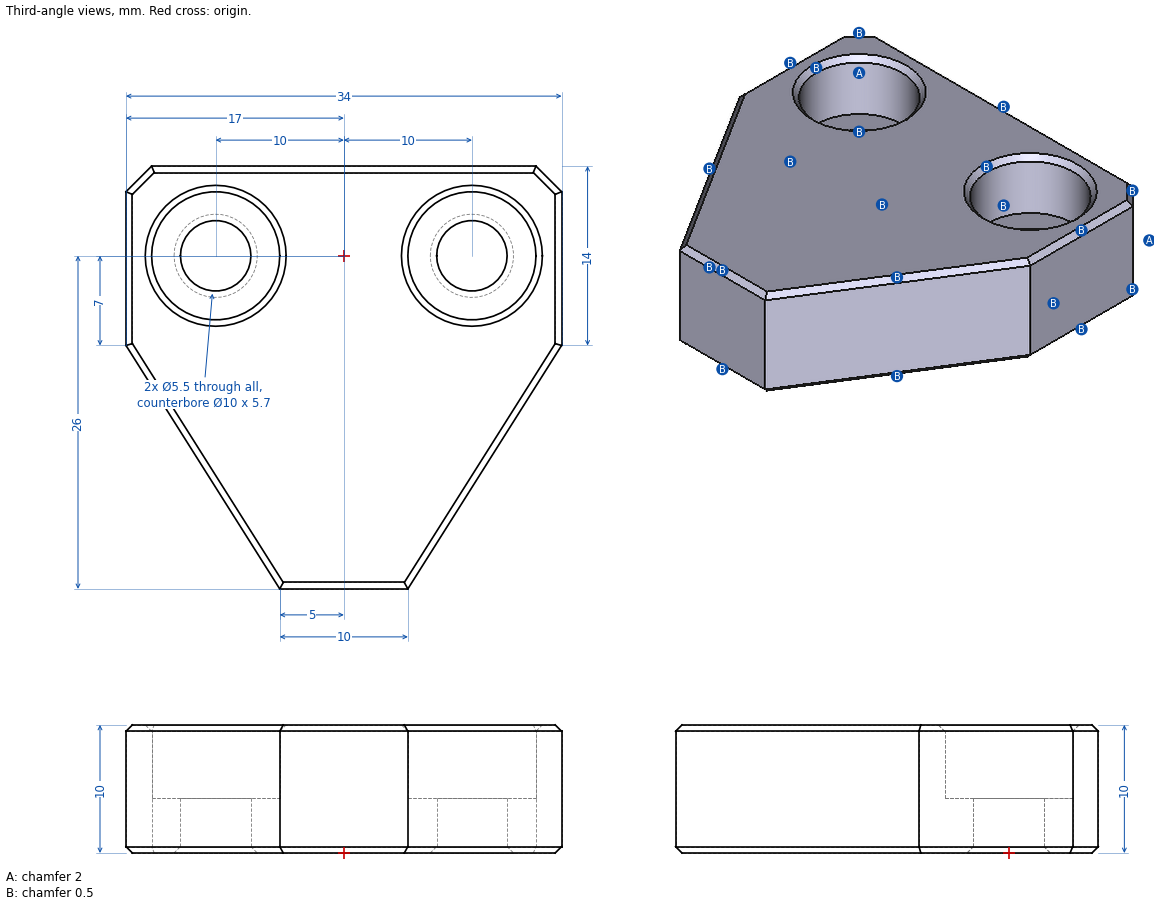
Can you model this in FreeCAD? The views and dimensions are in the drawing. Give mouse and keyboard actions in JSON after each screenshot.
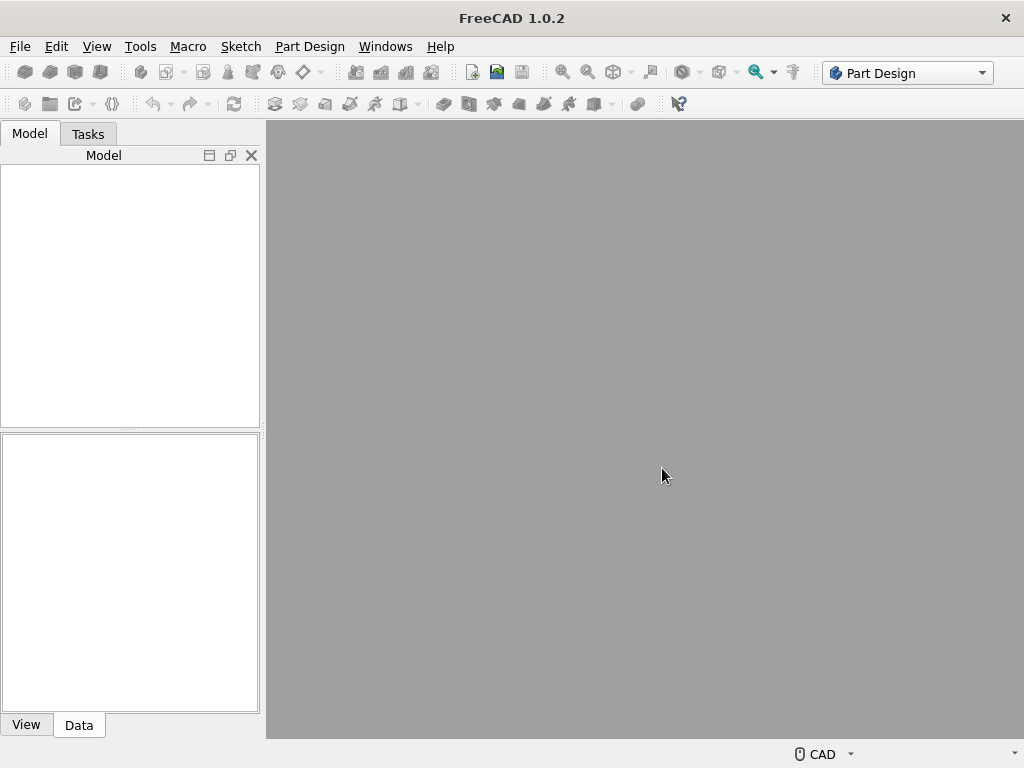
{"action": "left_click", "coordinate": [472, 72]}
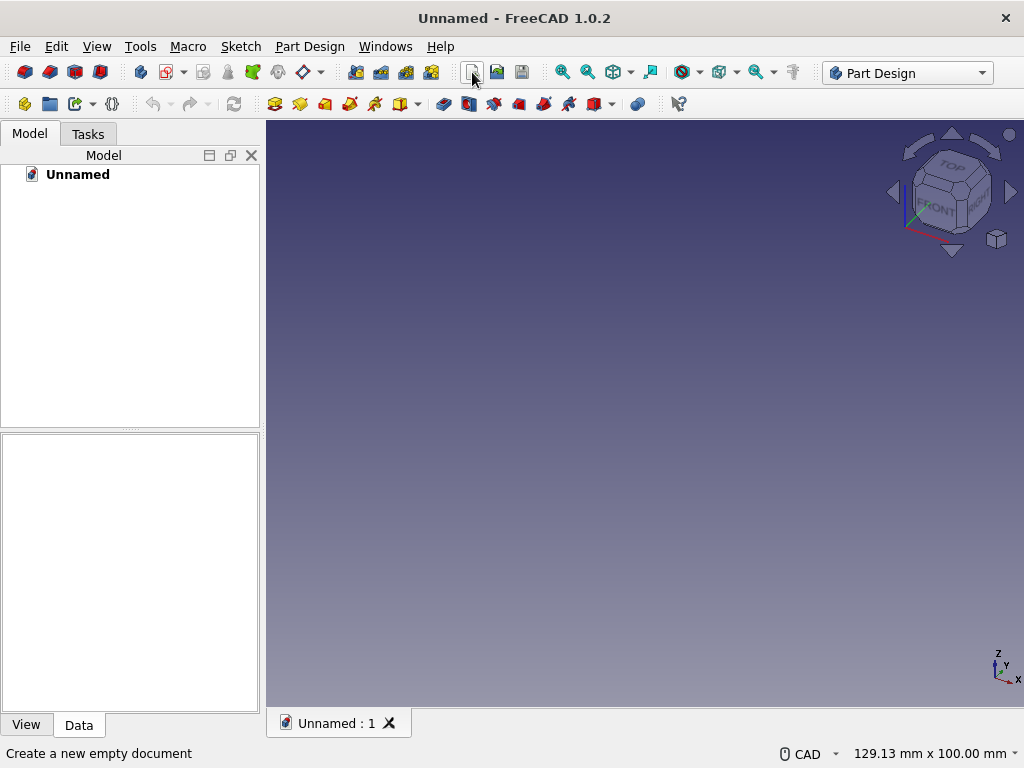
{"action": "left_click", "coordinate": [166, 72]}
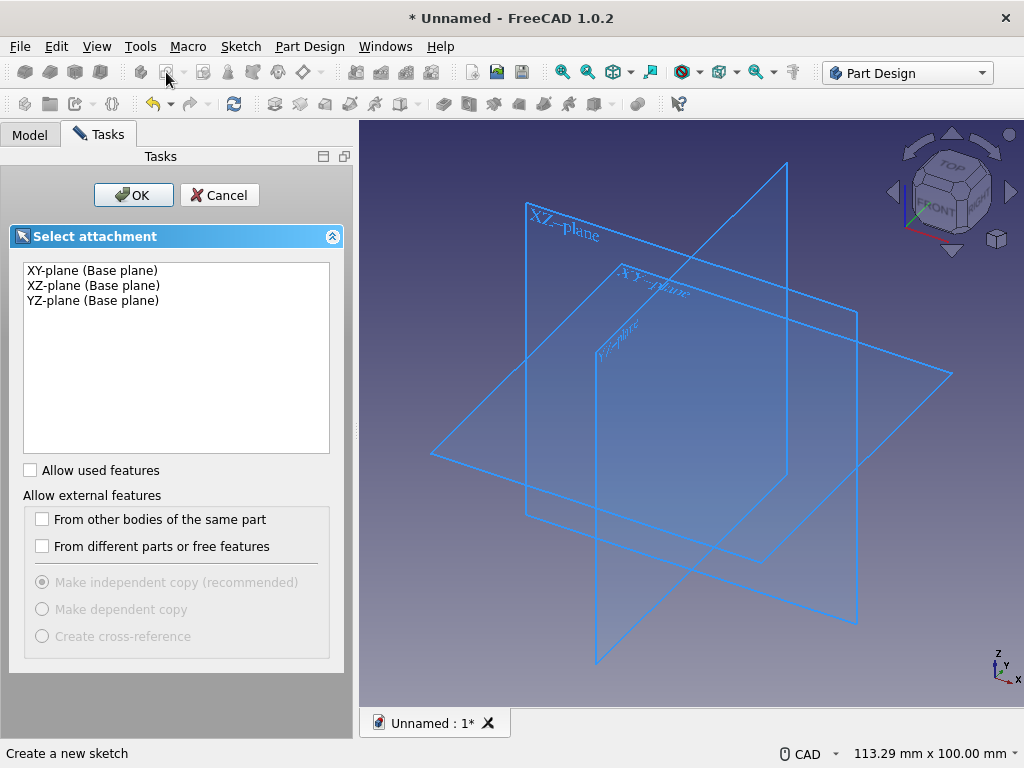
{"action": "left_click", "coordinate": [84, 270]}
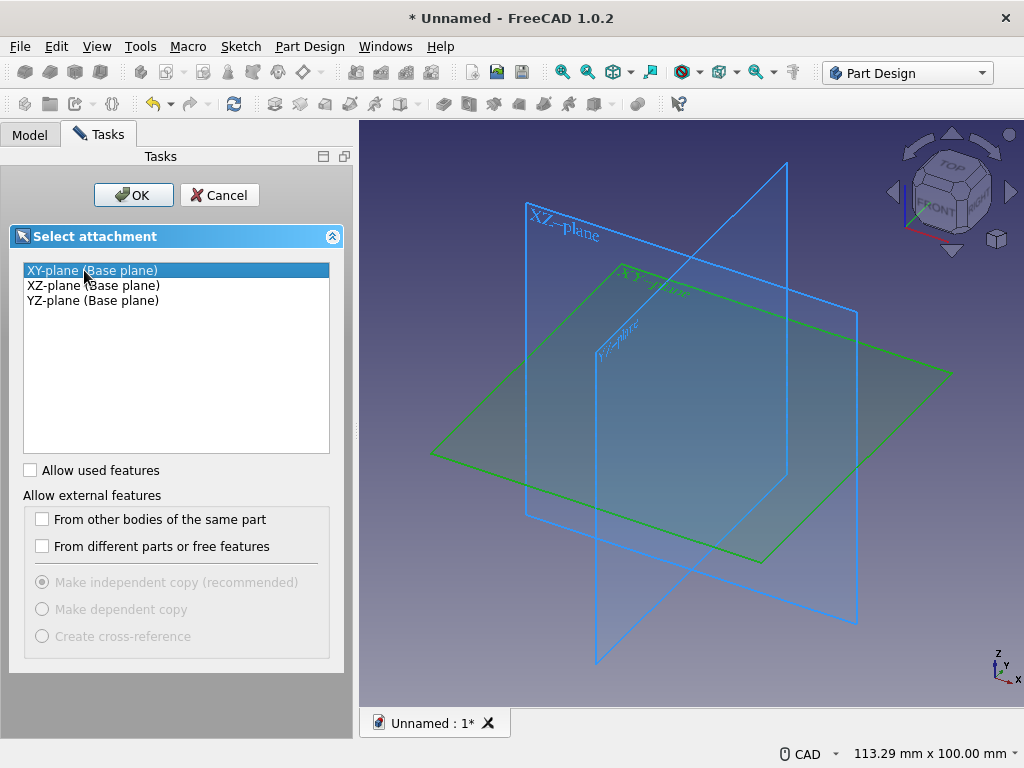
{"action": "left_click", "coordinate": [134, 195]}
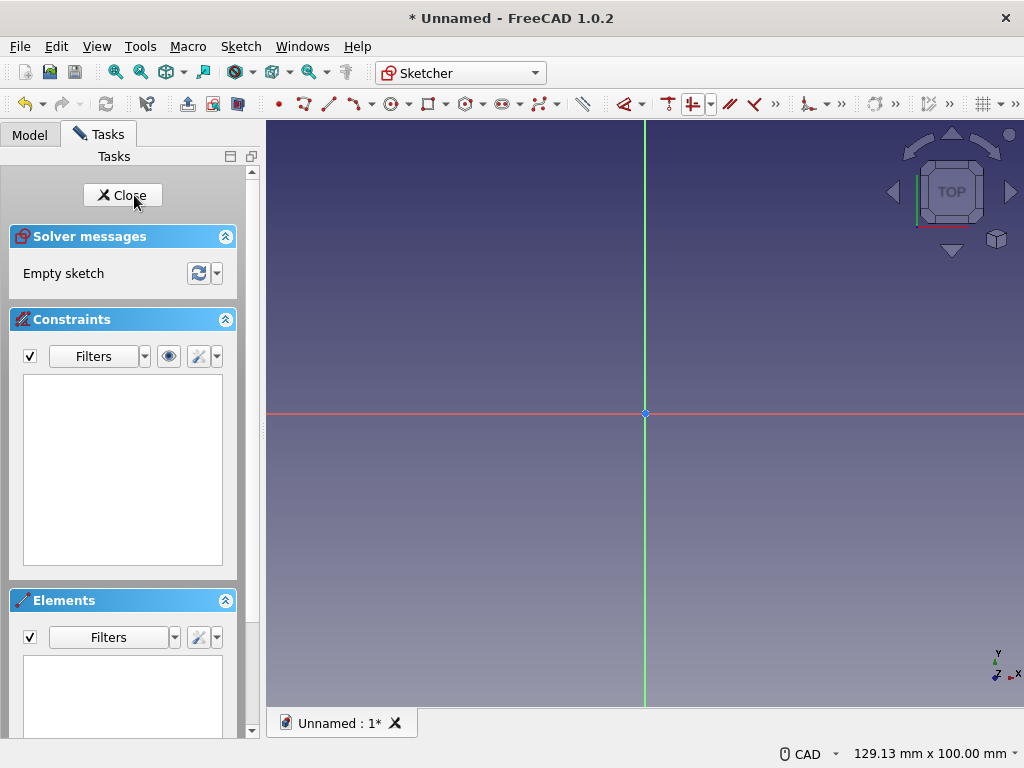
{"action": "scroll", "coordinate": [728, 414], "scroll_direction": "up", "scroll_amount": 3}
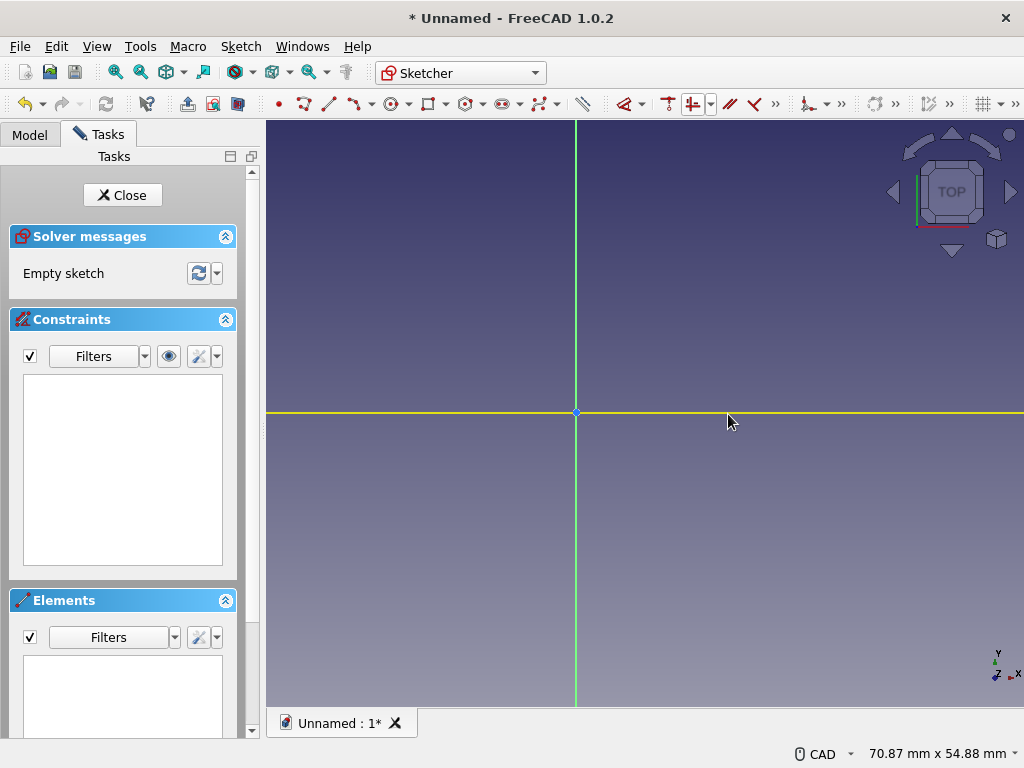
{"action": "key", "text": "g v"}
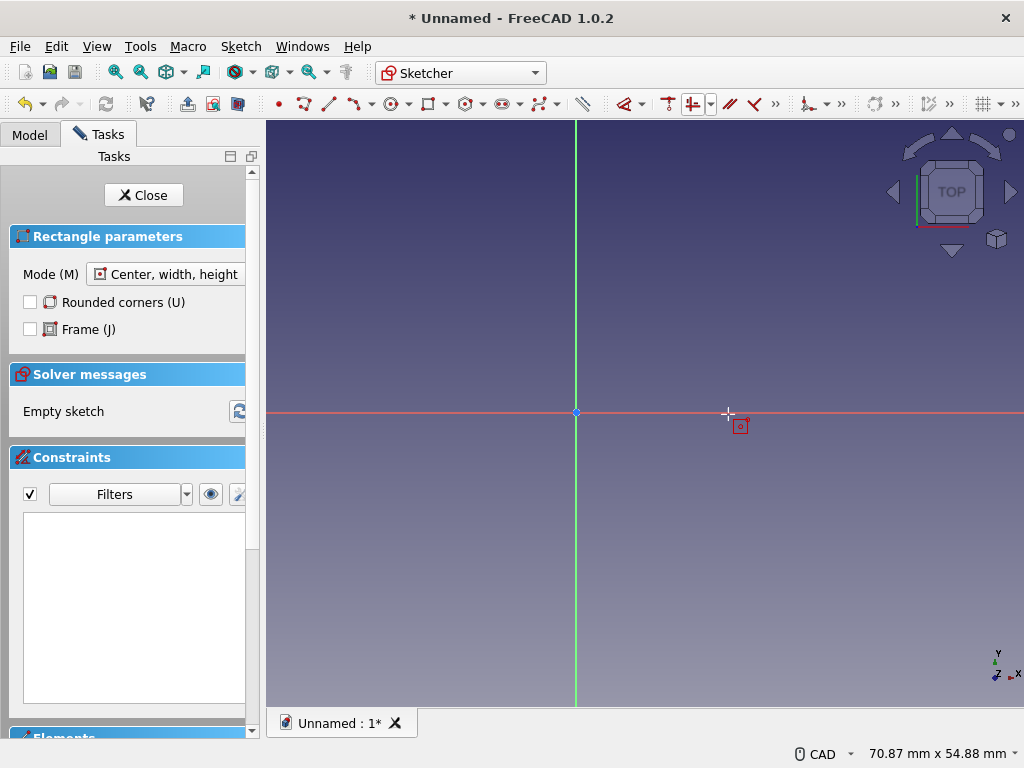
{"action": "left_click", "coordinate": [576, 413]}
{"action": "mouse_move", "coordinate": [758, 338]}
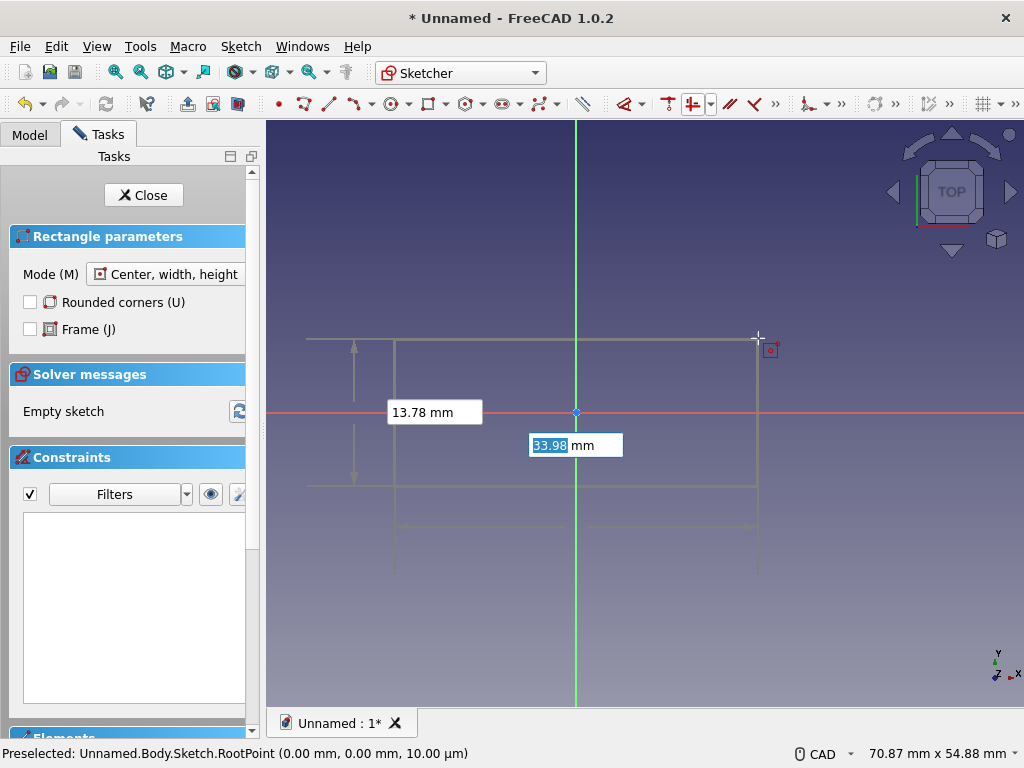
{"action": "type", "text": "34"}
{"action": "key", "text": "Tab"}
{"action": "type", "text": "14"}
{"action": "key", "text": "Return"}
{"action": "key", "text": "Escape"}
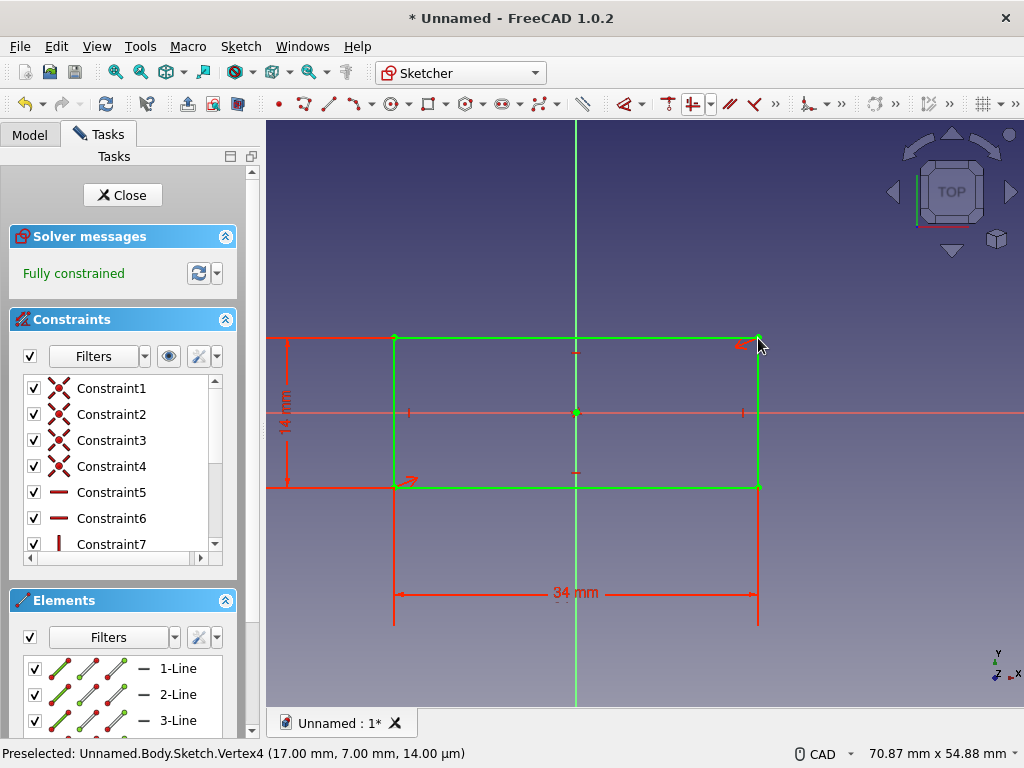
{"action": "left_click", "coordinate": [123, 195]}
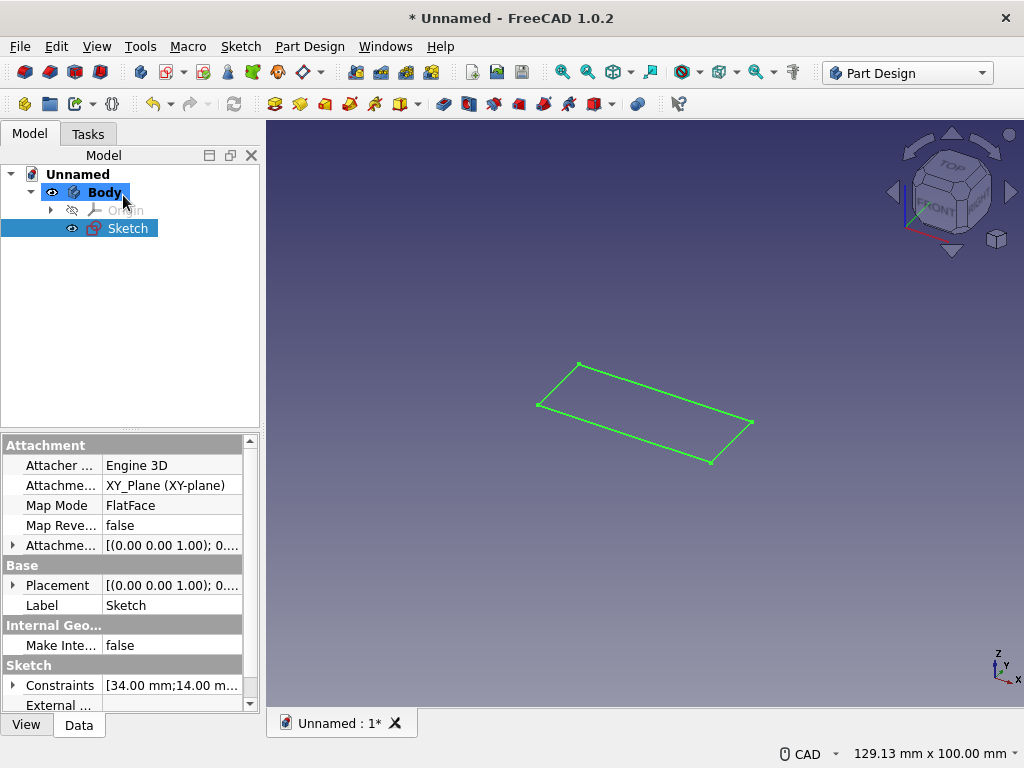
{"action": "left_click", "coordinate": [275, 104]}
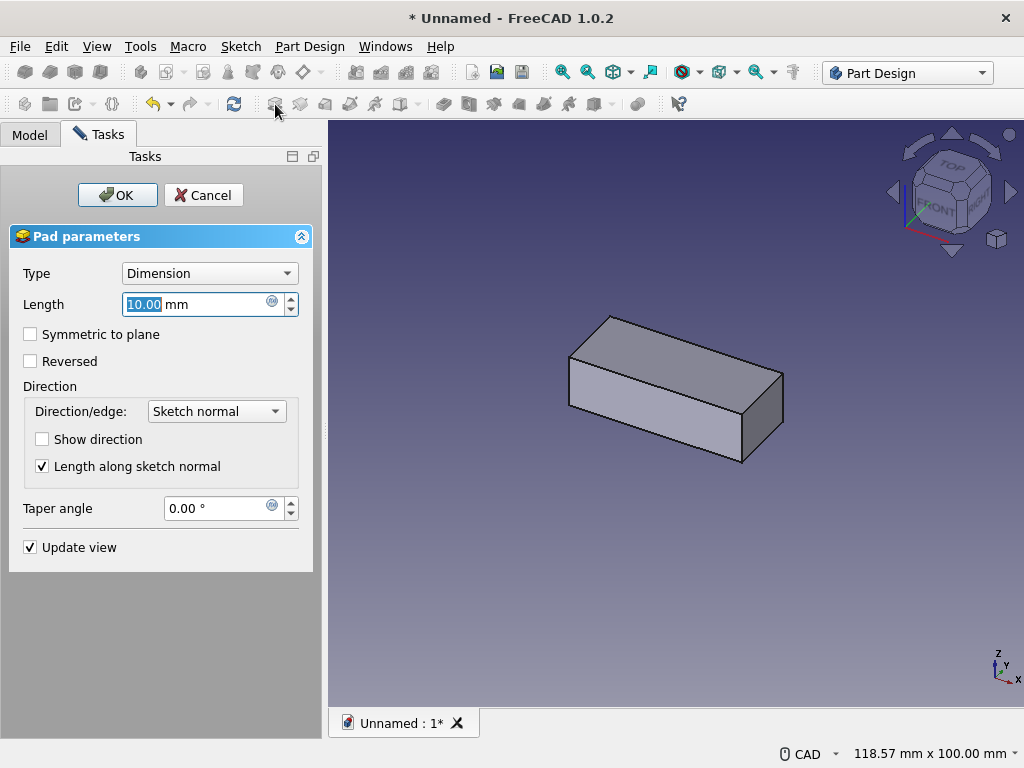
{"action": "type", "text": "10"}
{"action": "key", "text": "Tab"}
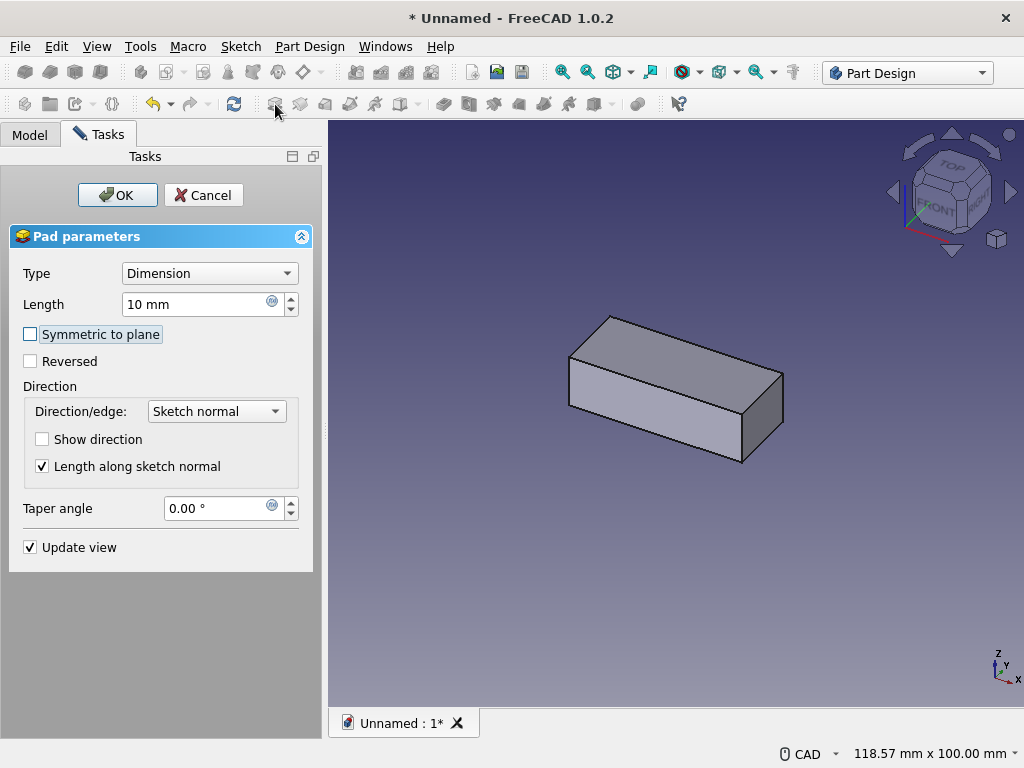
{"action": "left_click", "coordinate": [118, 195]}